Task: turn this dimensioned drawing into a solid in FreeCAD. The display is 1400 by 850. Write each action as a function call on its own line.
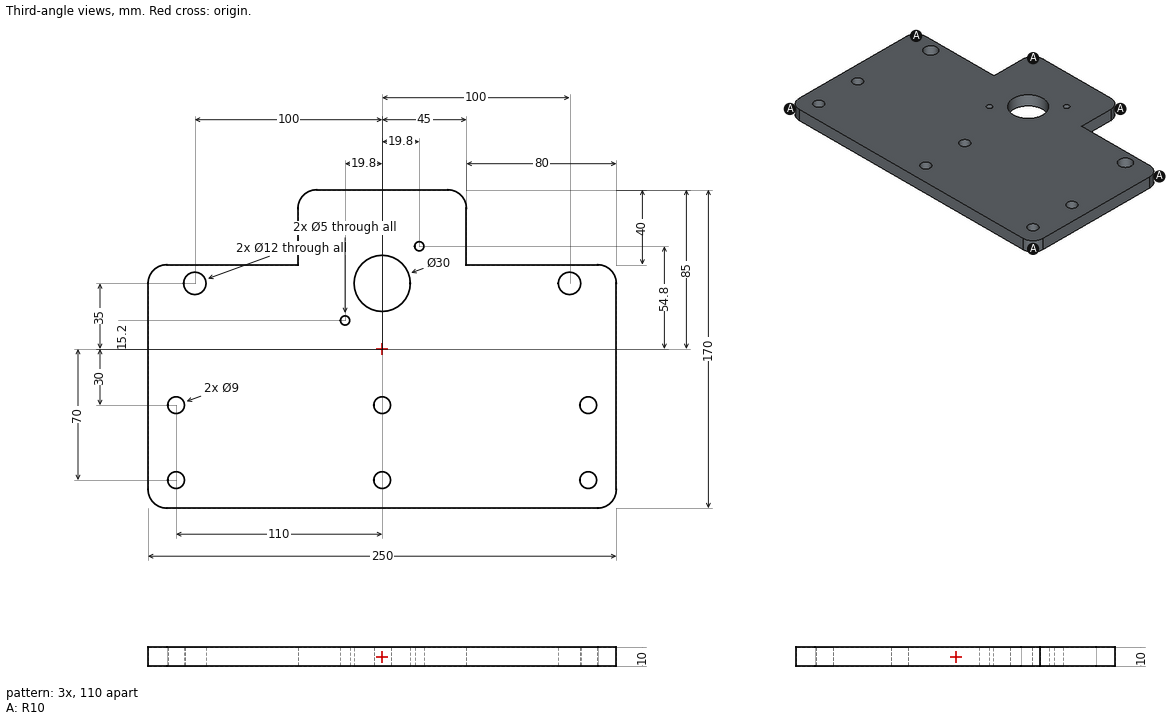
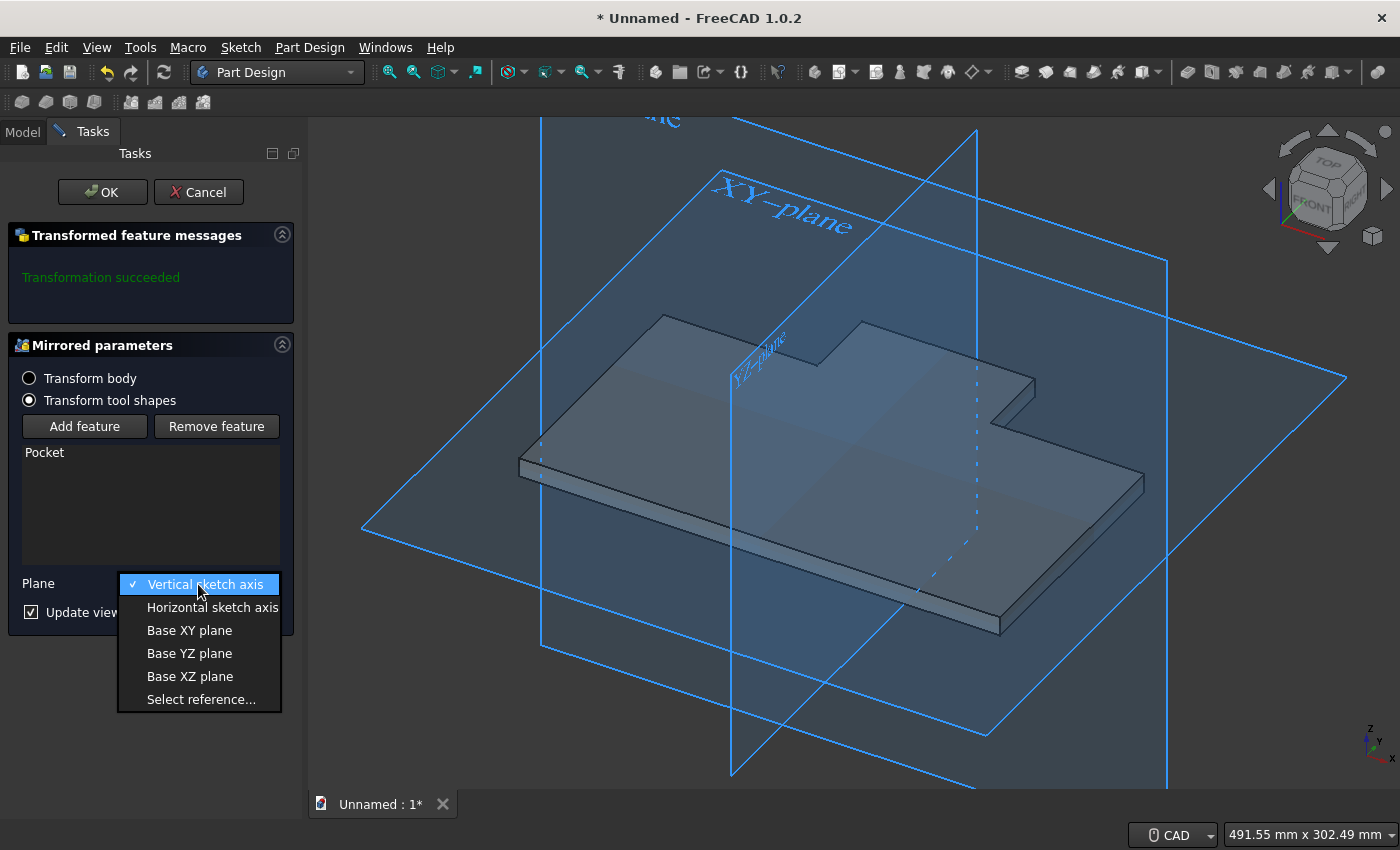
click(198, 654)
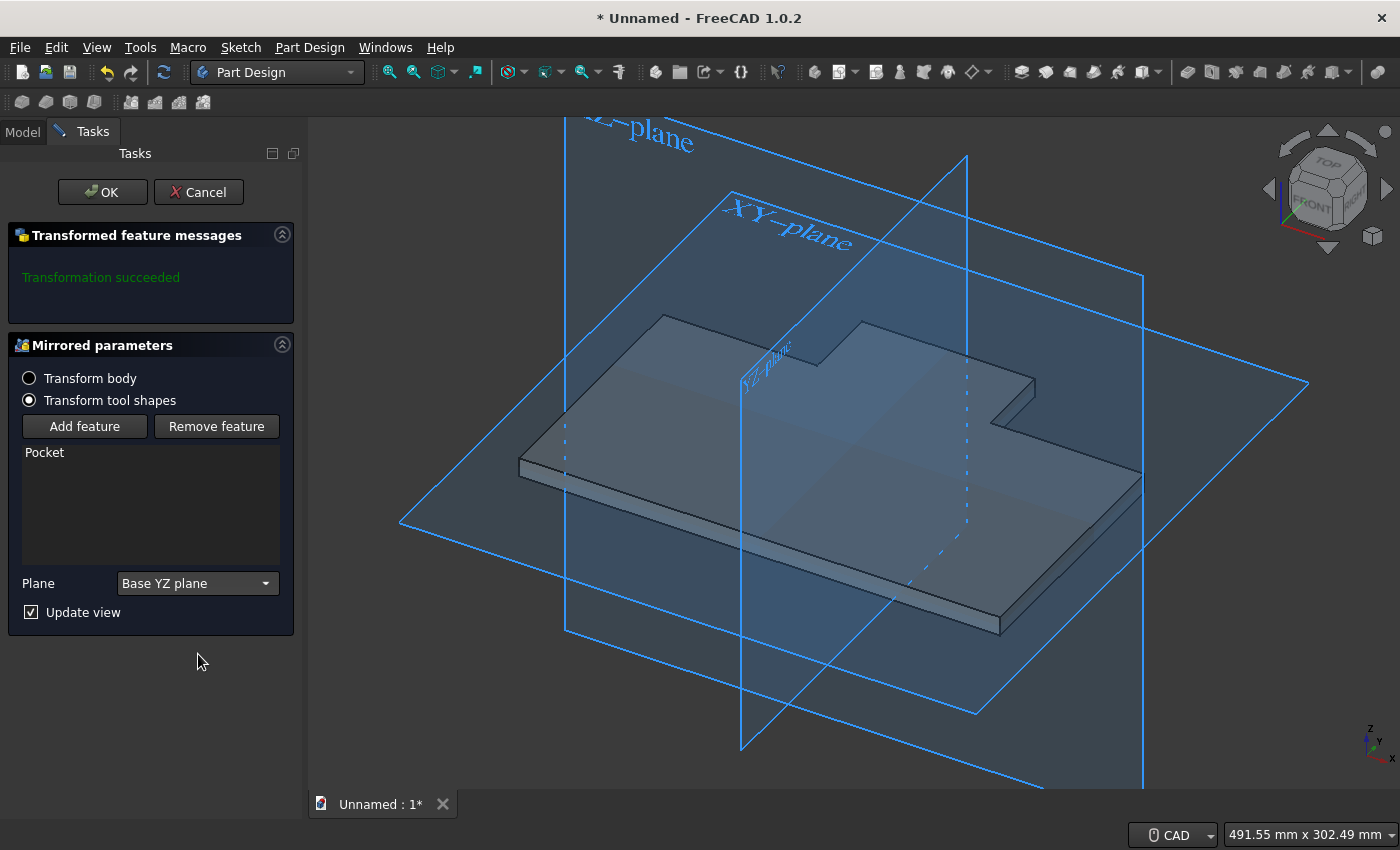
click(103, 192)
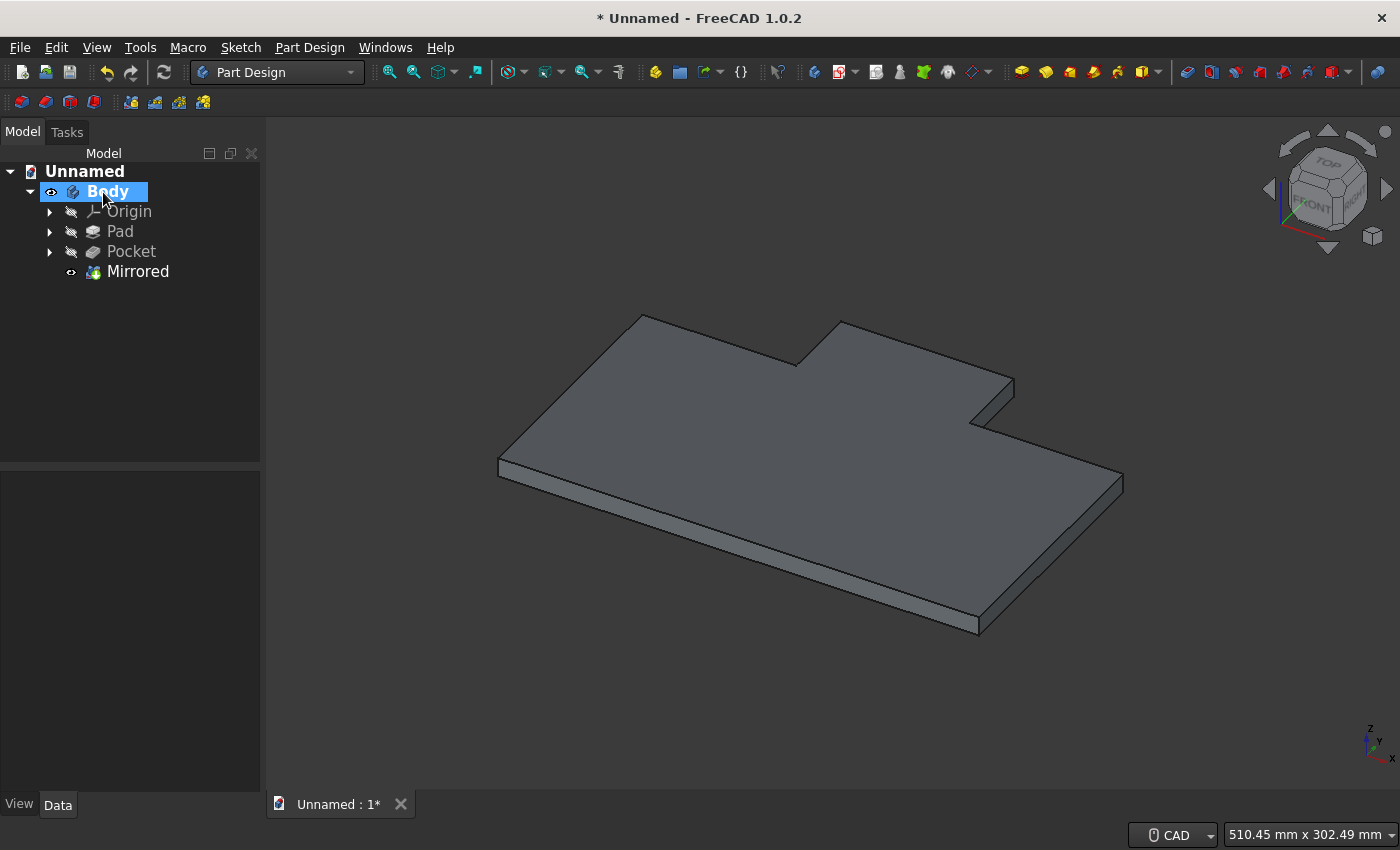
click(833, 443)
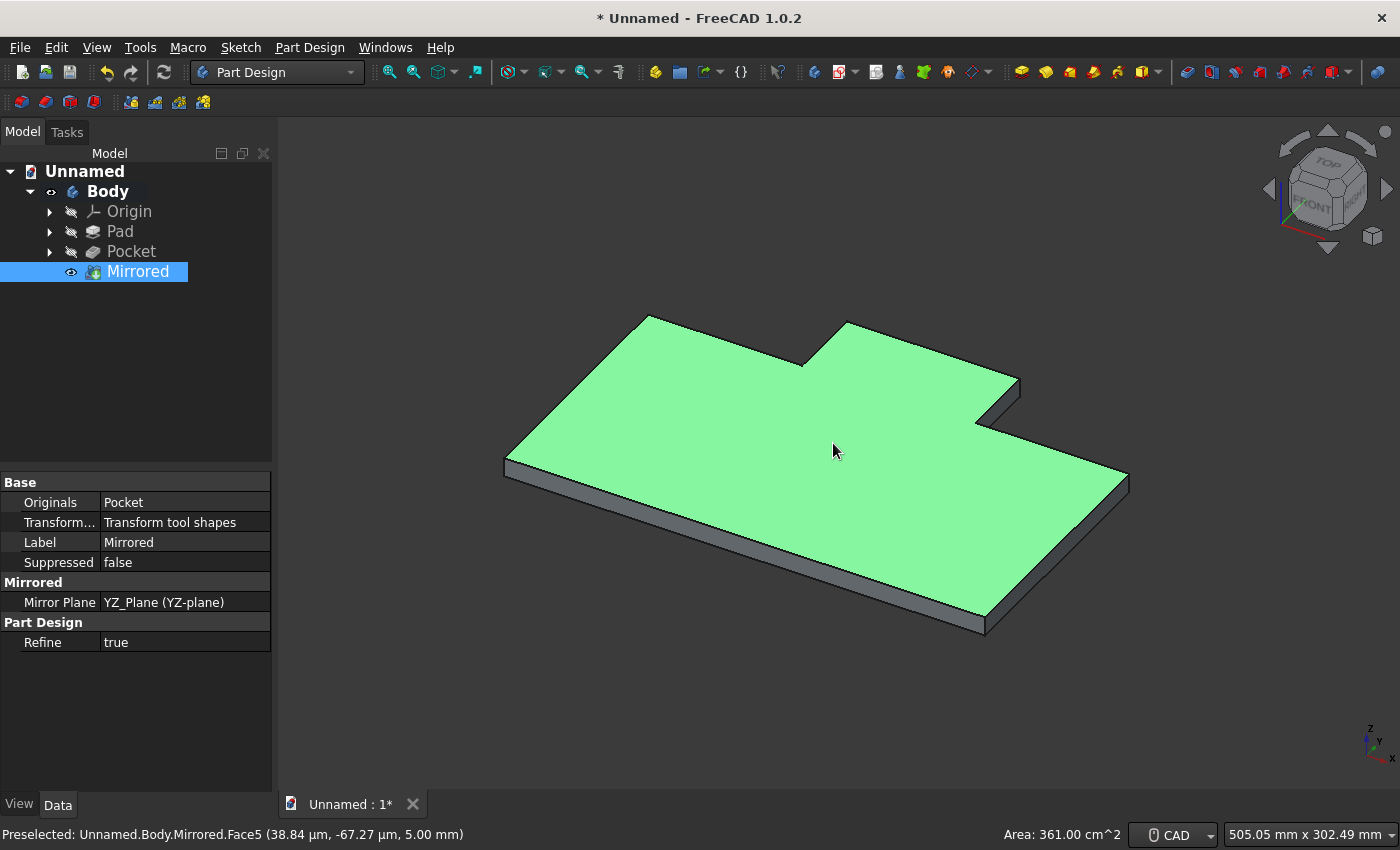
click(840, 72)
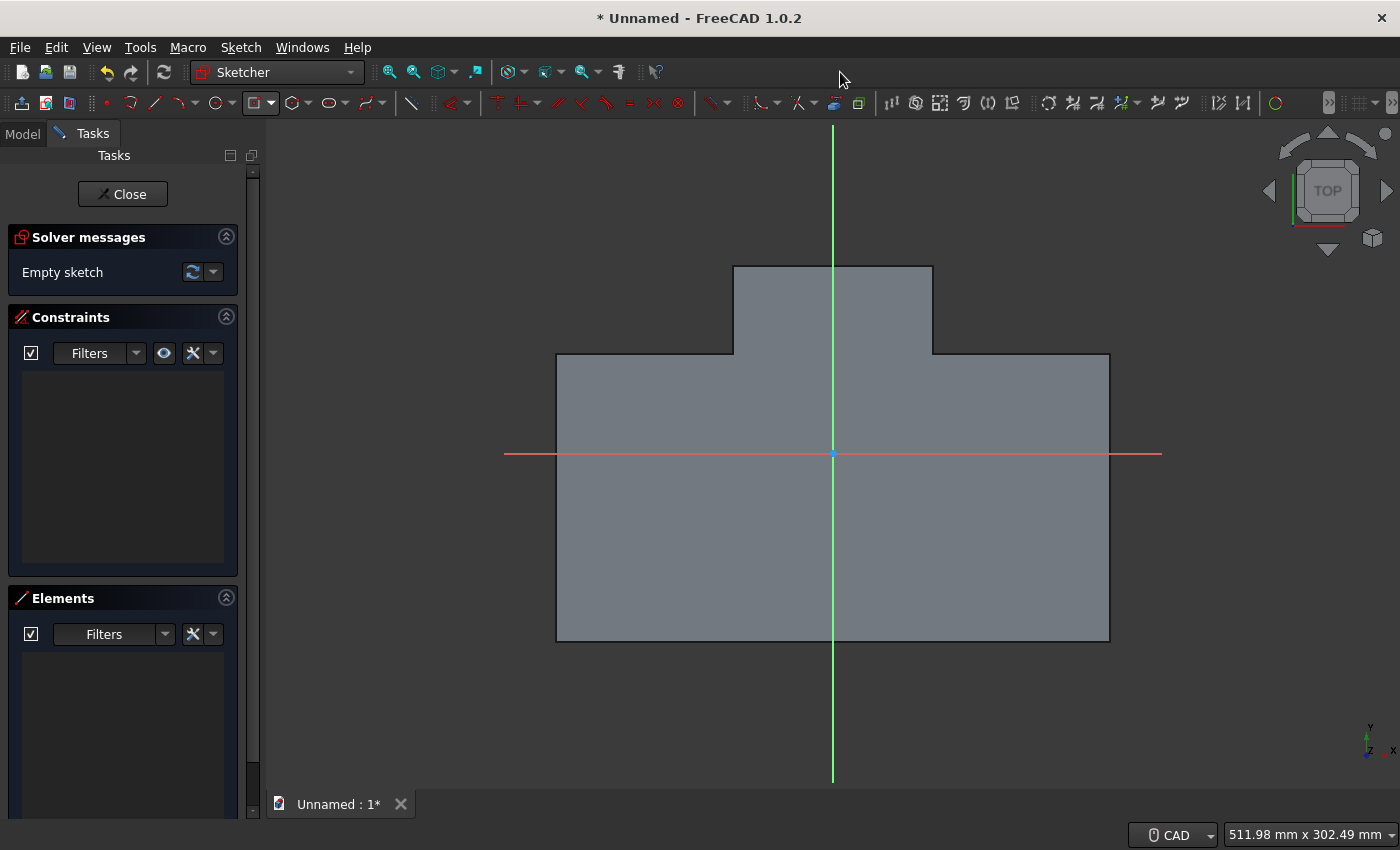
scroll(672, 585, up, 5)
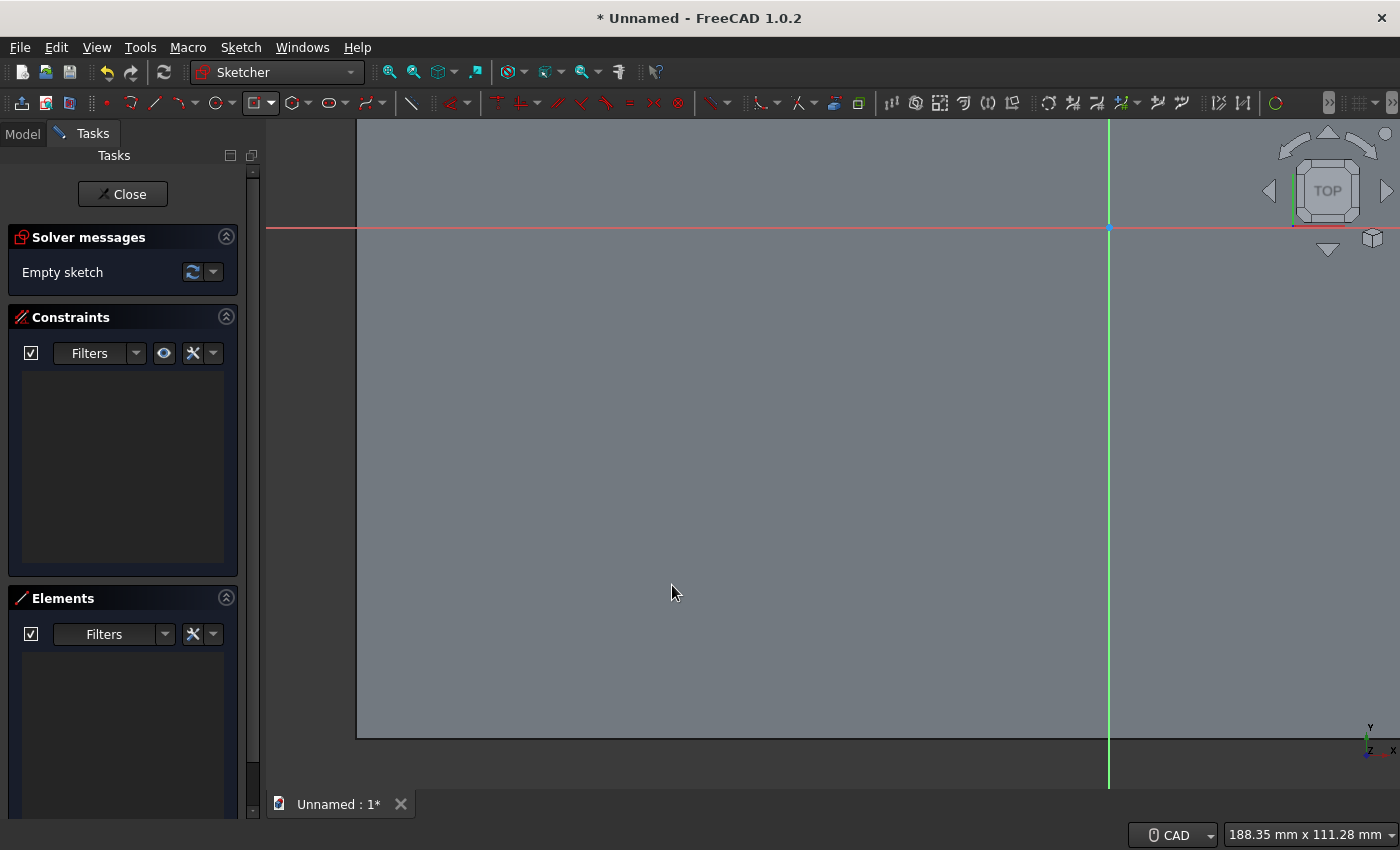
click(216, 104)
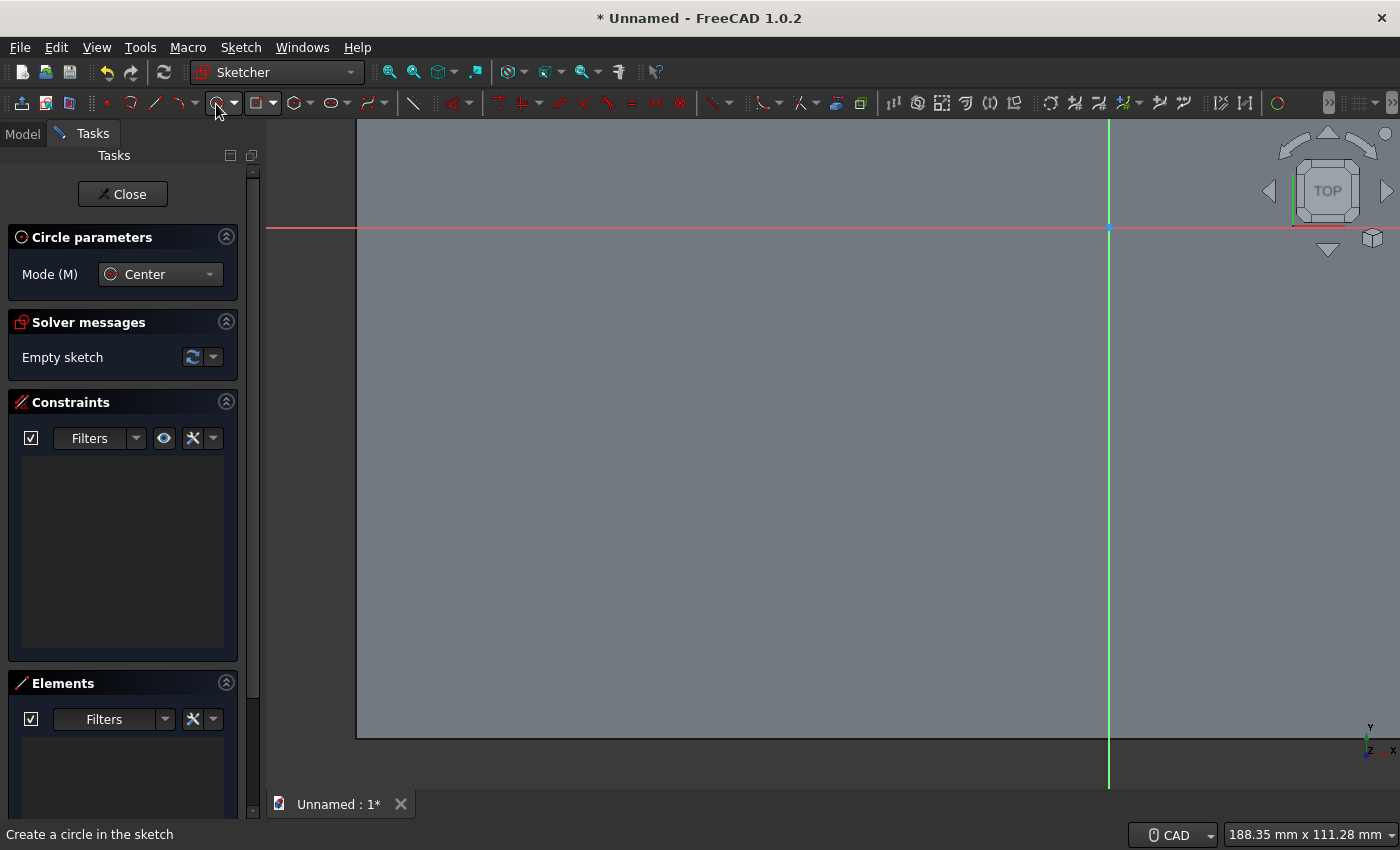
click(447, 408)
move(466, 389)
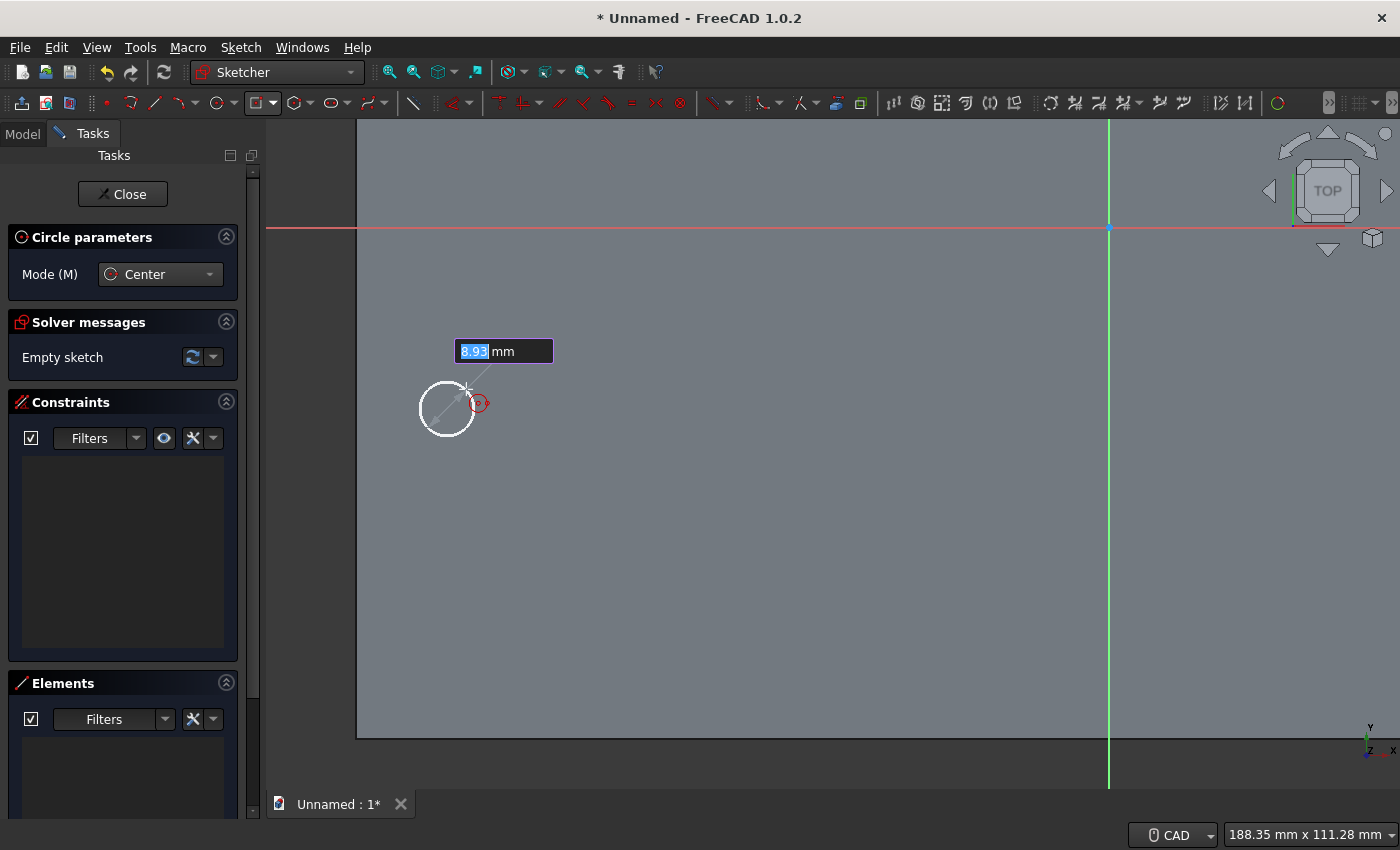
text(9)
key(Return)